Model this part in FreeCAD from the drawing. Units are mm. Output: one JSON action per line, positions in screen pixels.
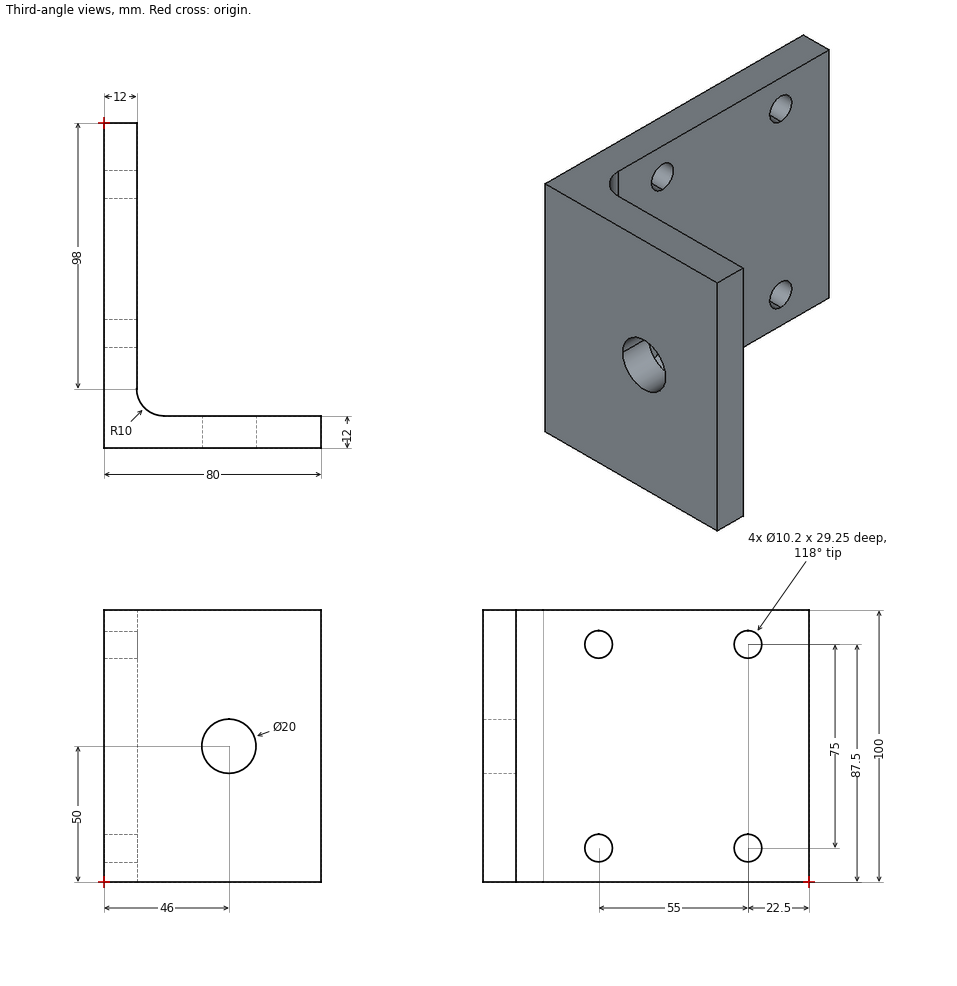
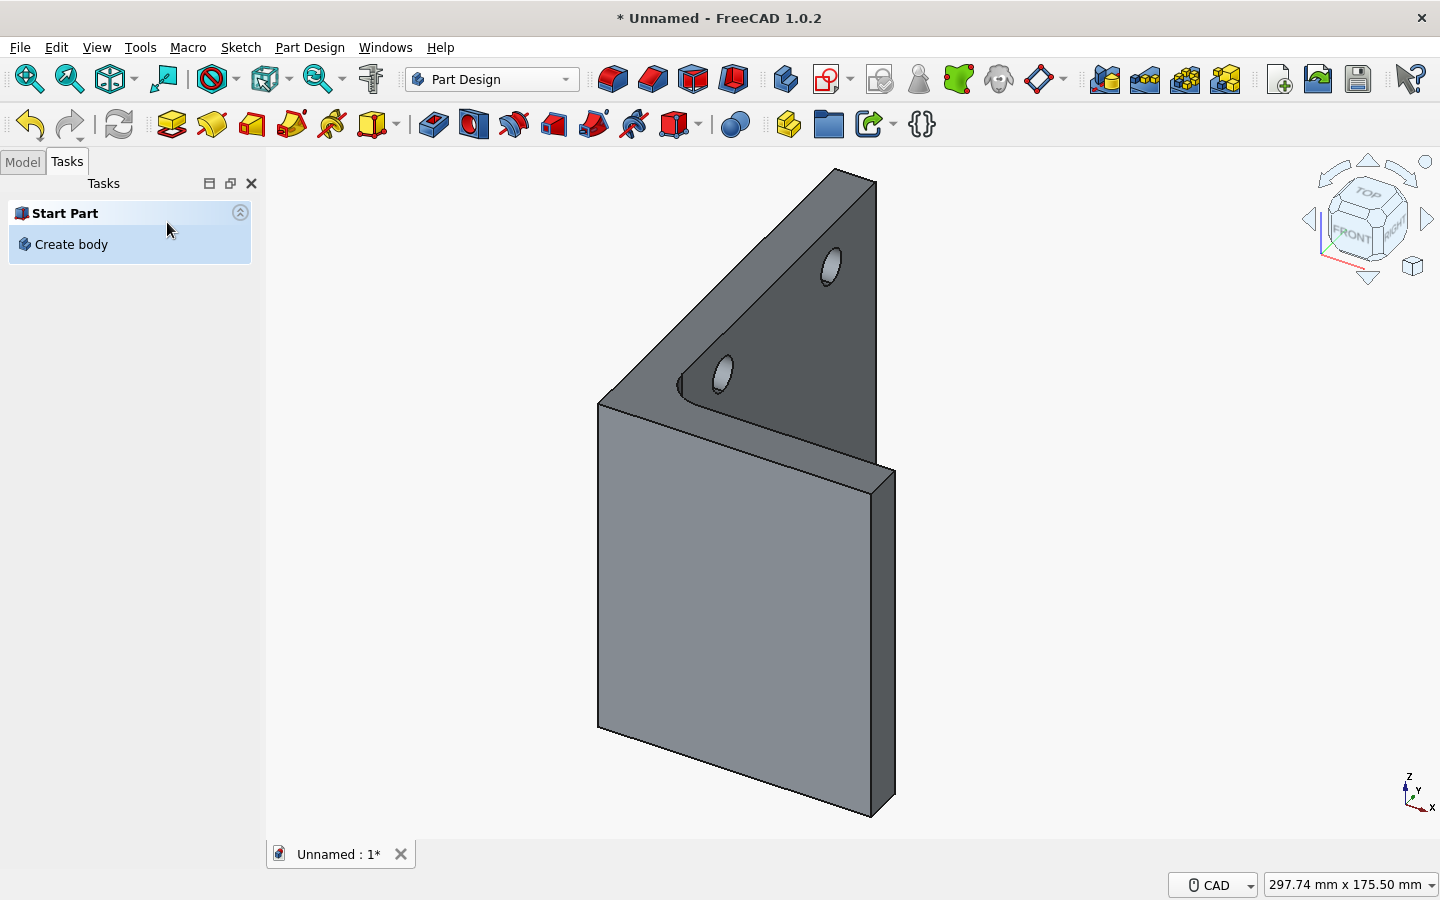
{"action": "key", "text": "4"}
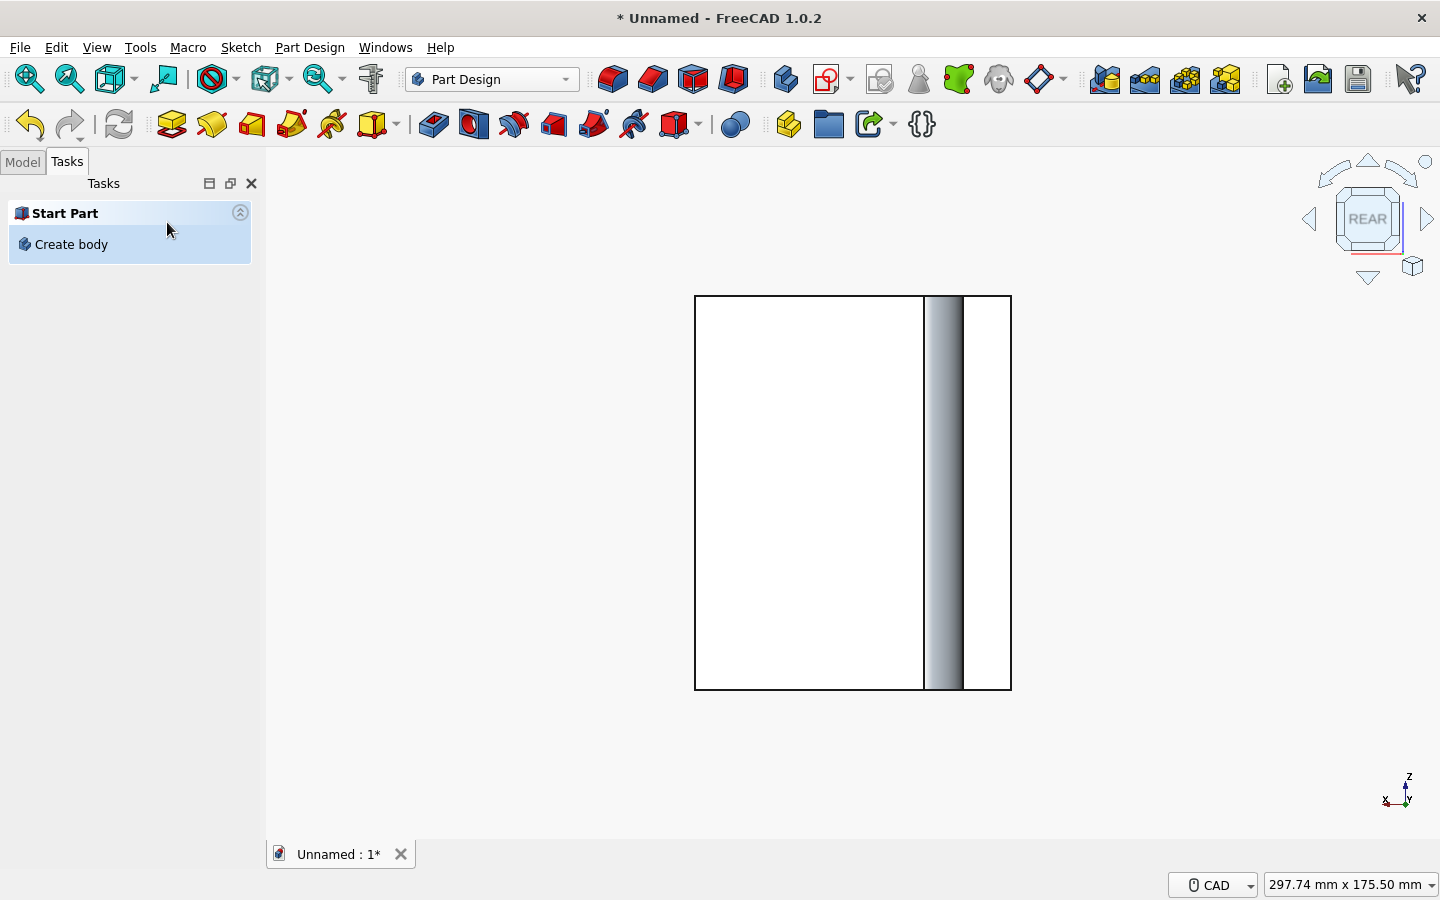
{"action": "left_click", "coordinate": [810, 436]}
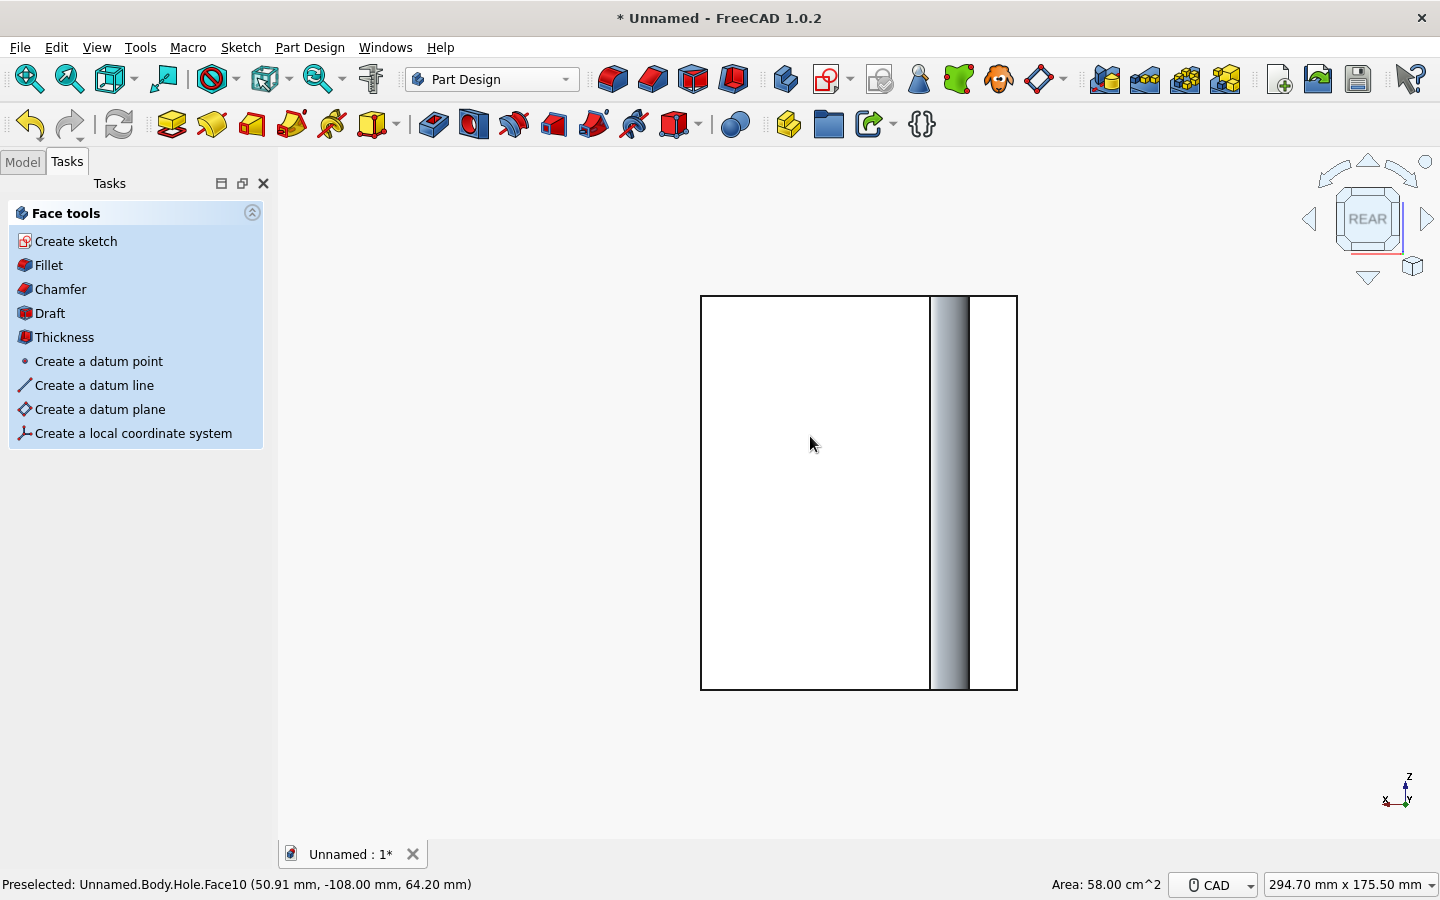
{"action": "left_click", "coordinate": [826, 80]}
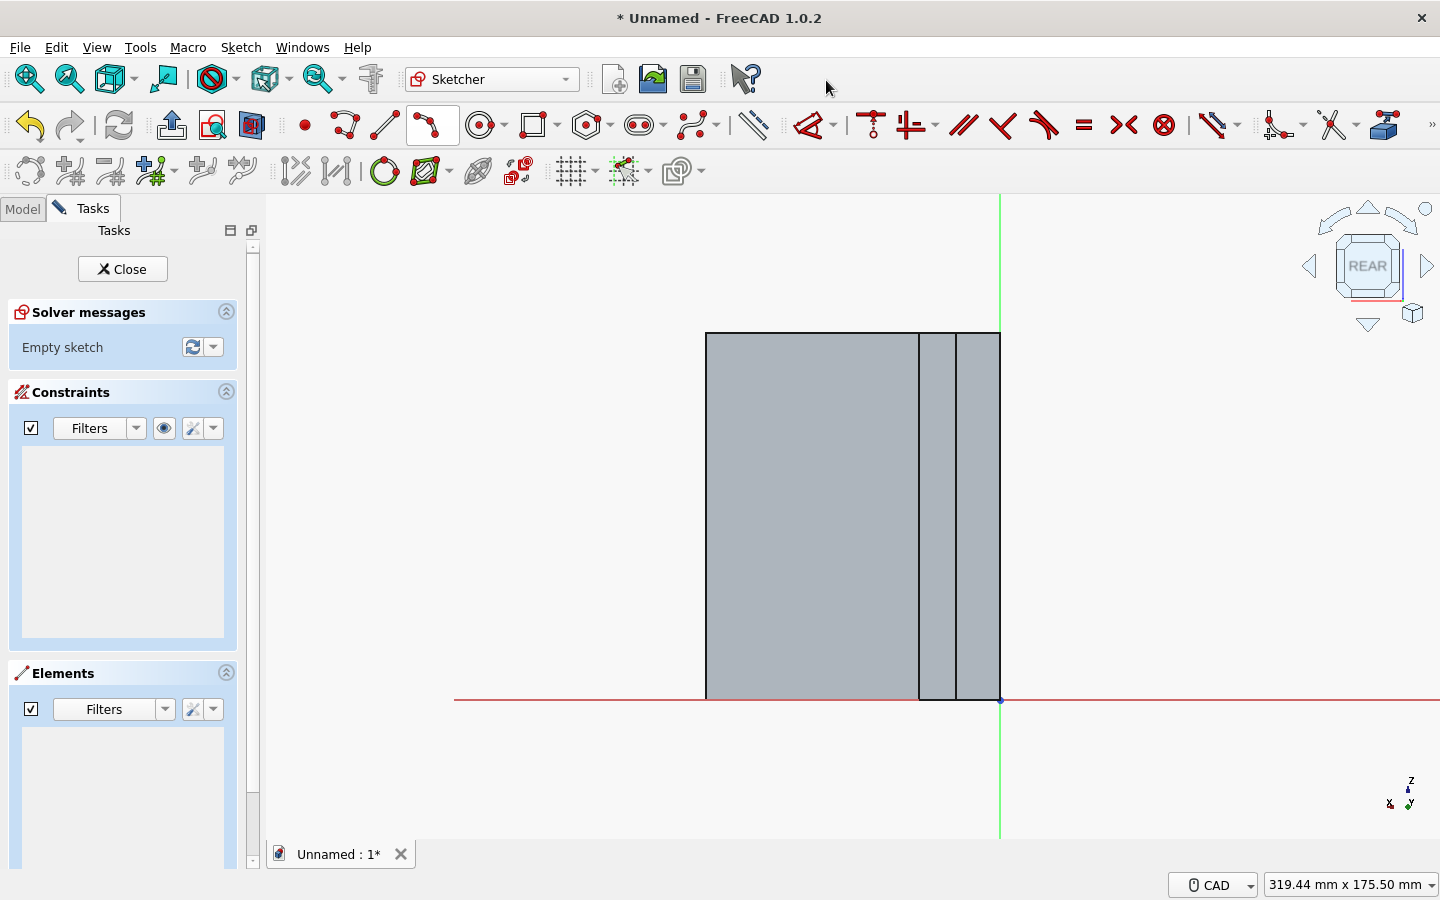
{"action": "key", "text": "q s"}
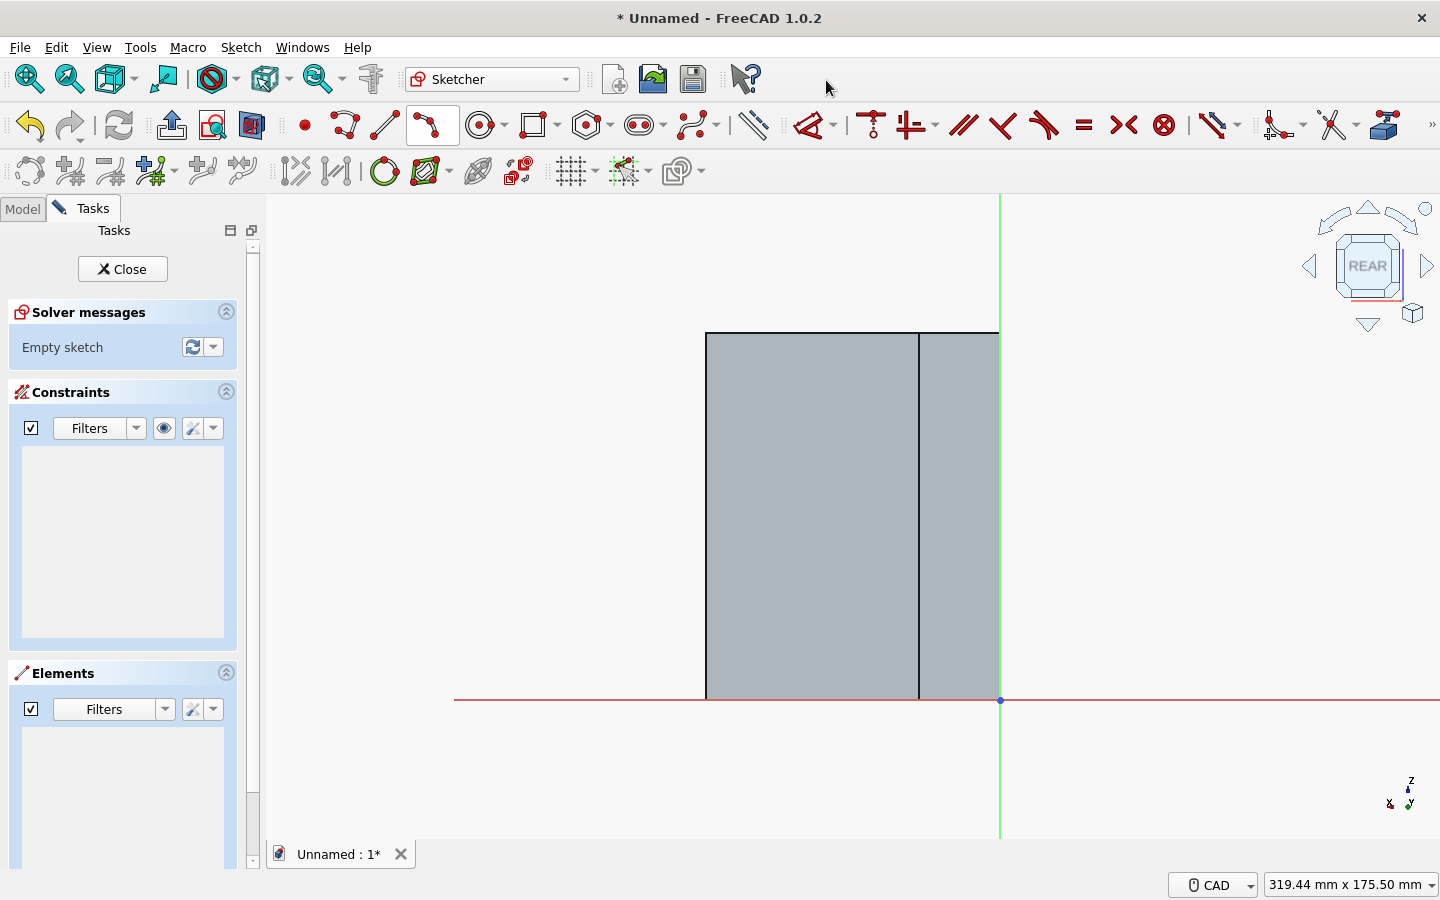
{"action": "scroll", "coordinate": [840, 516], "scroll_direction": "up", "scroll_amount": 9}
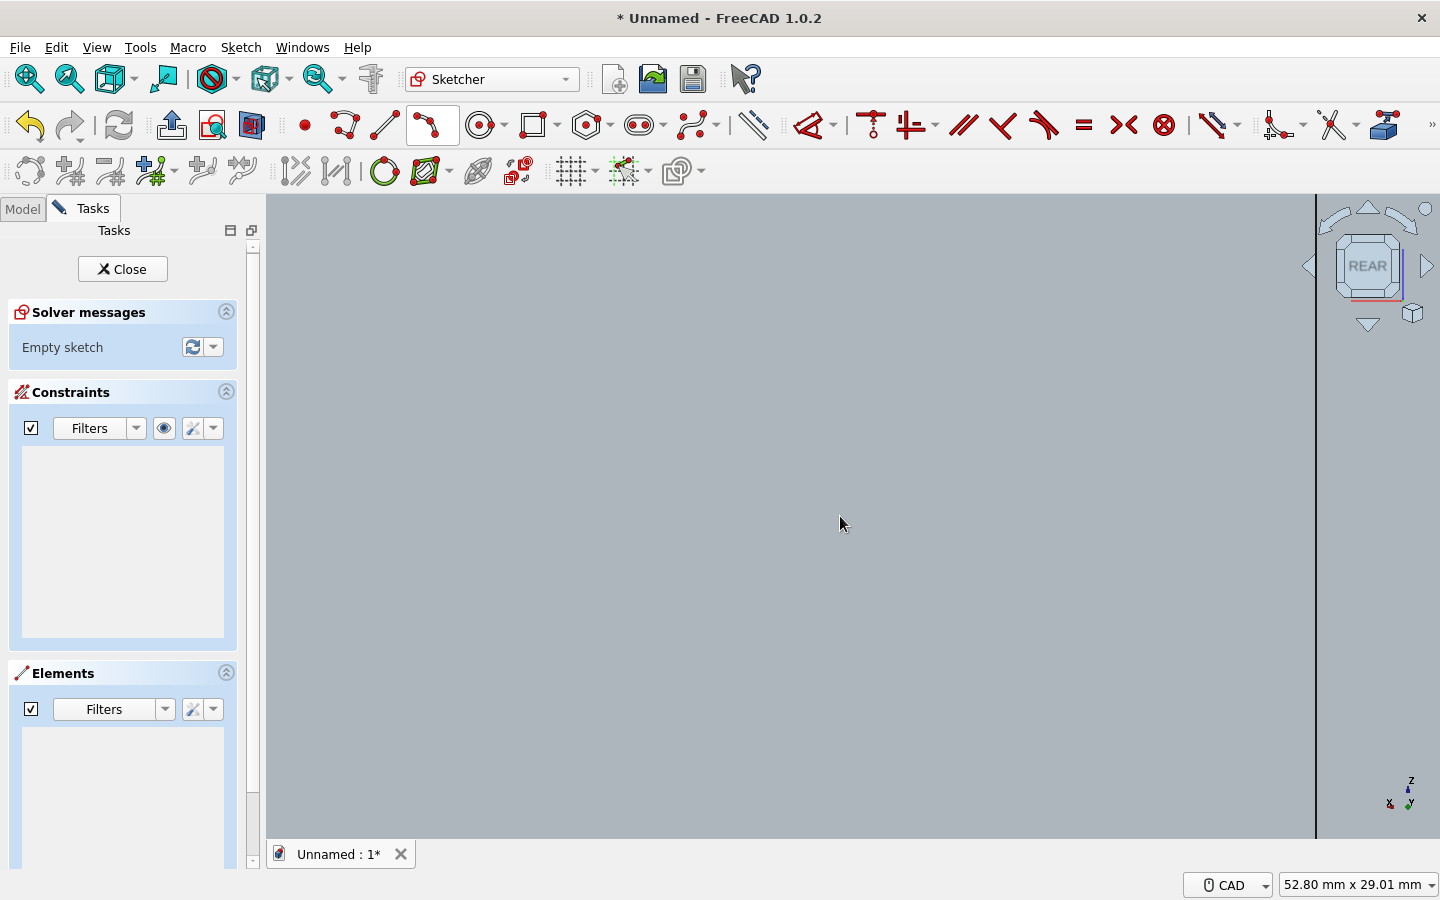
{"action": "key", "text": "g c"}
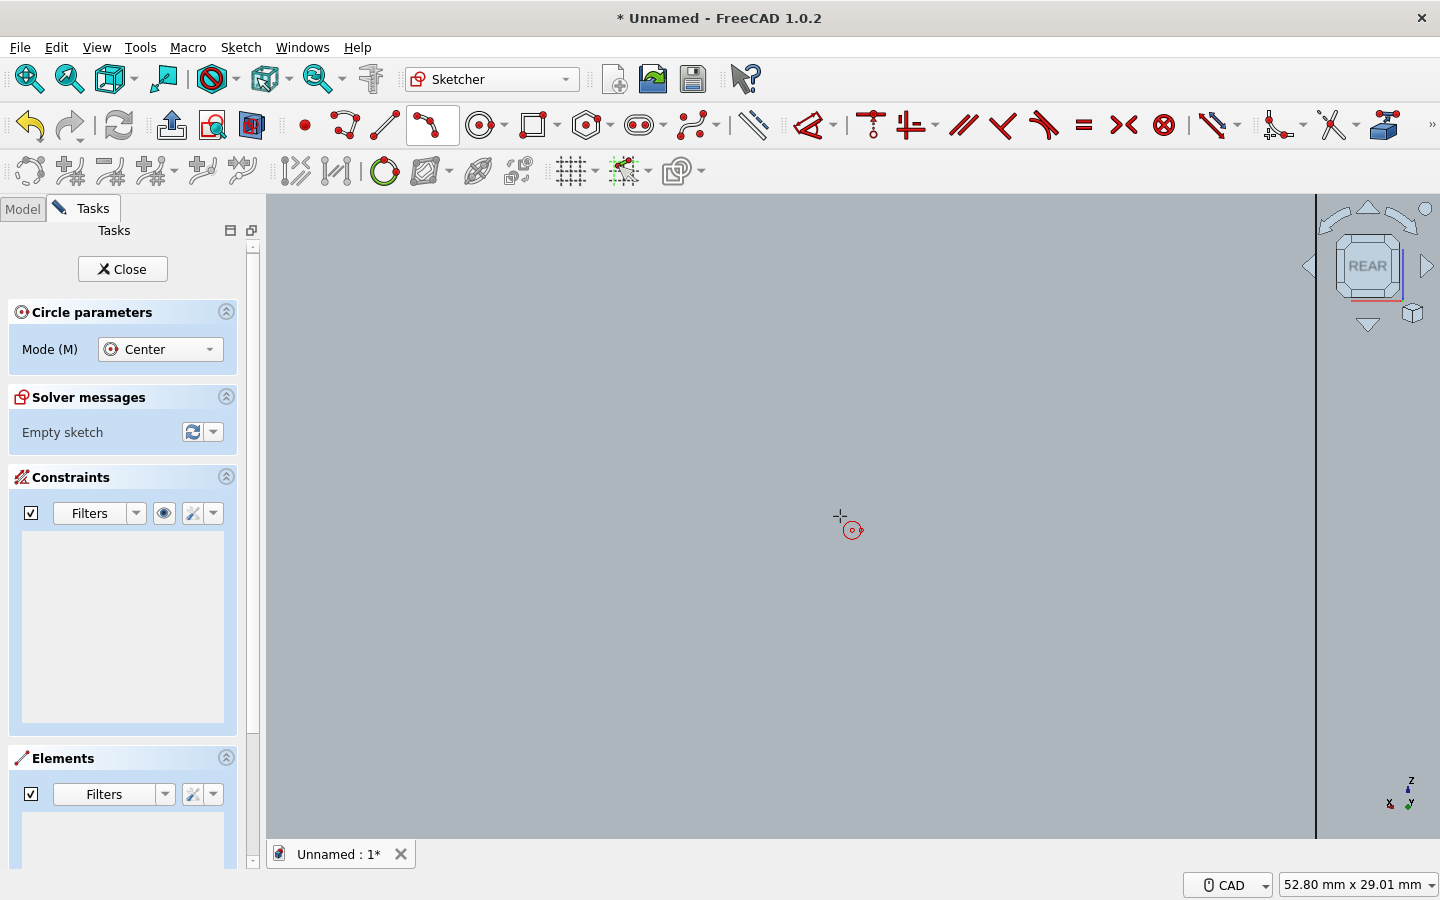
{"action": "left_click", "coordinate": [783, 516]}
{"action": "mouse_move", "coordinate": [940, 359]}